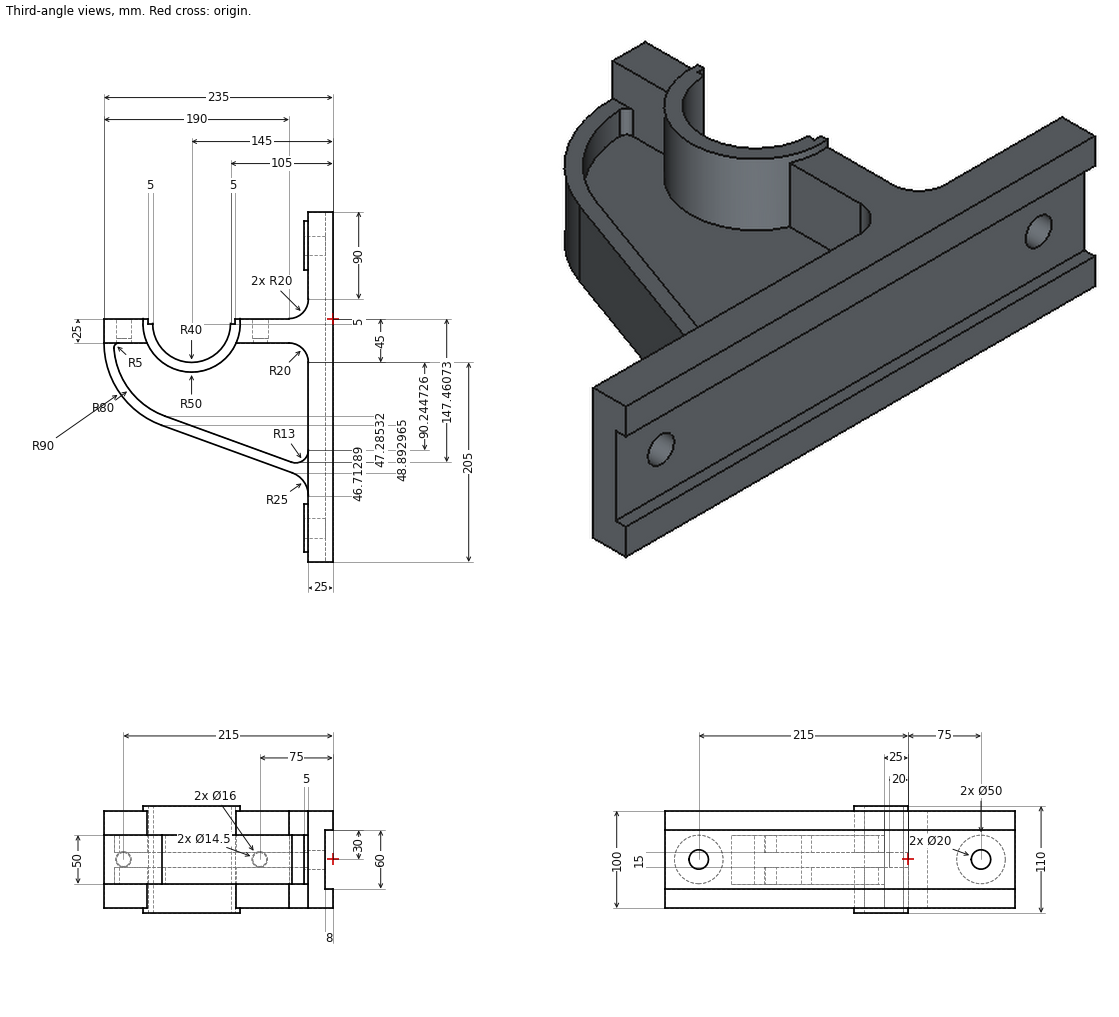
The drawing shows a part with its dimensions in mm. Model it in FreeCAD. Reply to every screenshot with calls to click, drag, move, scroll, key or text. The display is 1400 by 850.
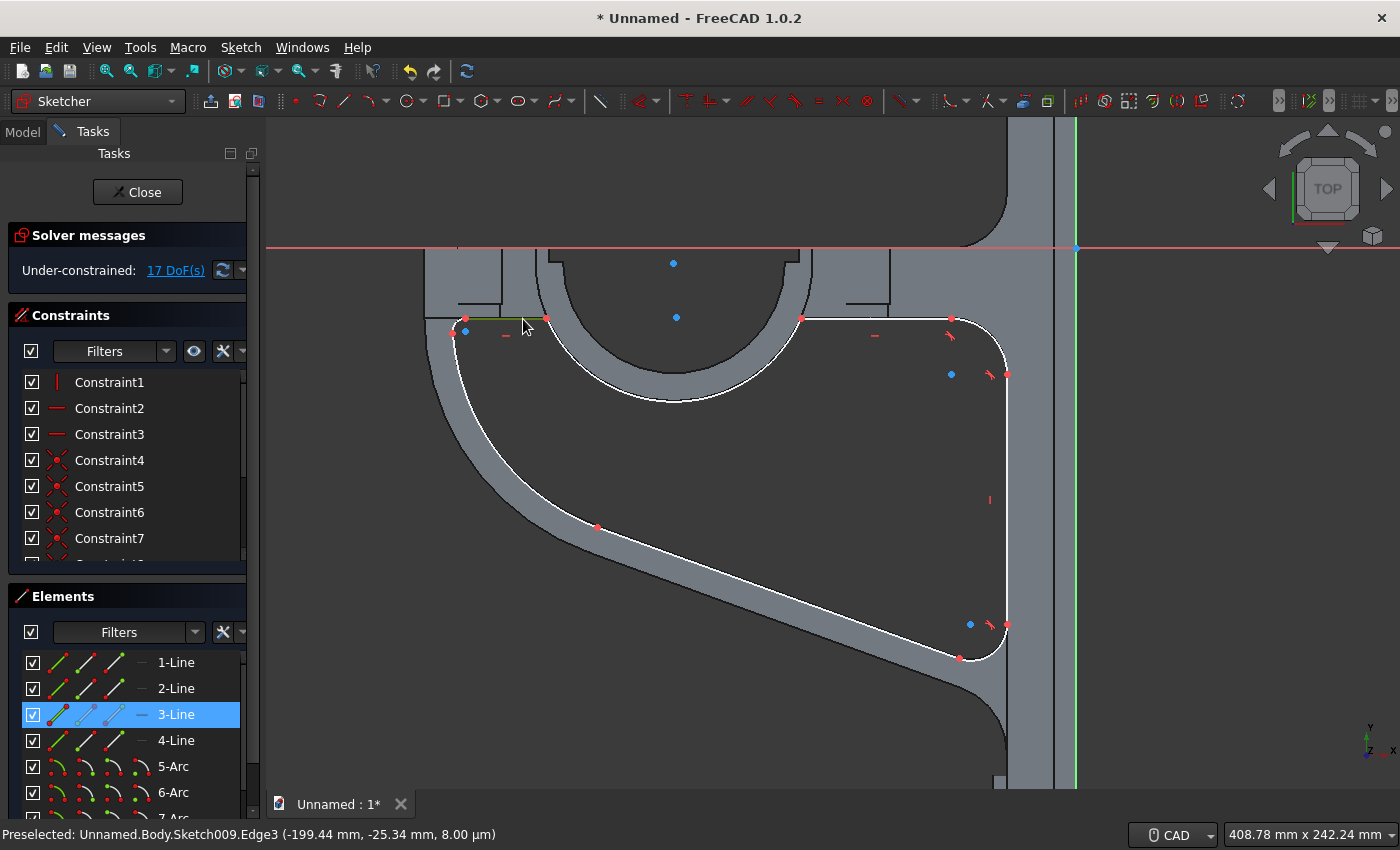
scroll(456, 323, up, 2)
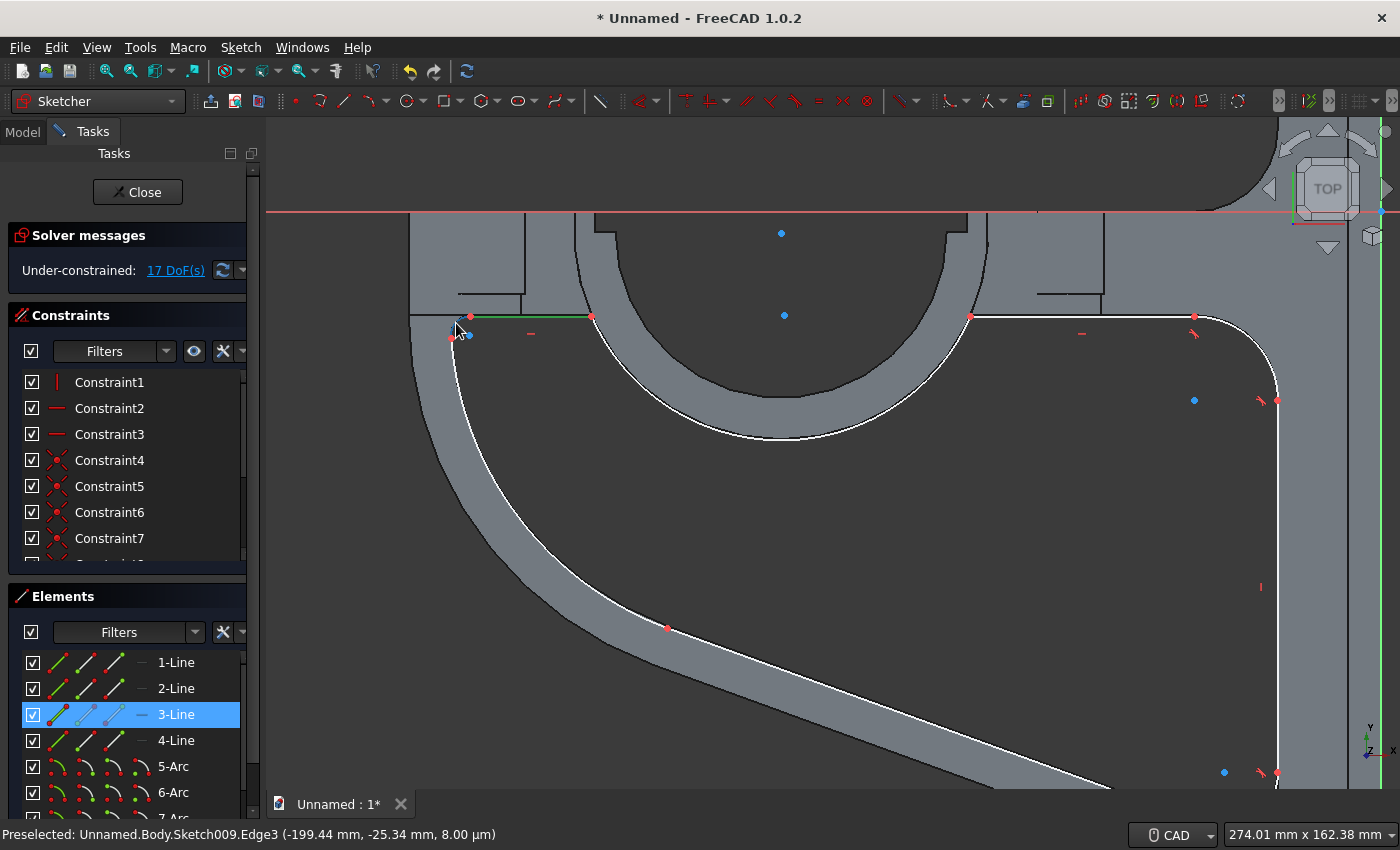
click(456, 323)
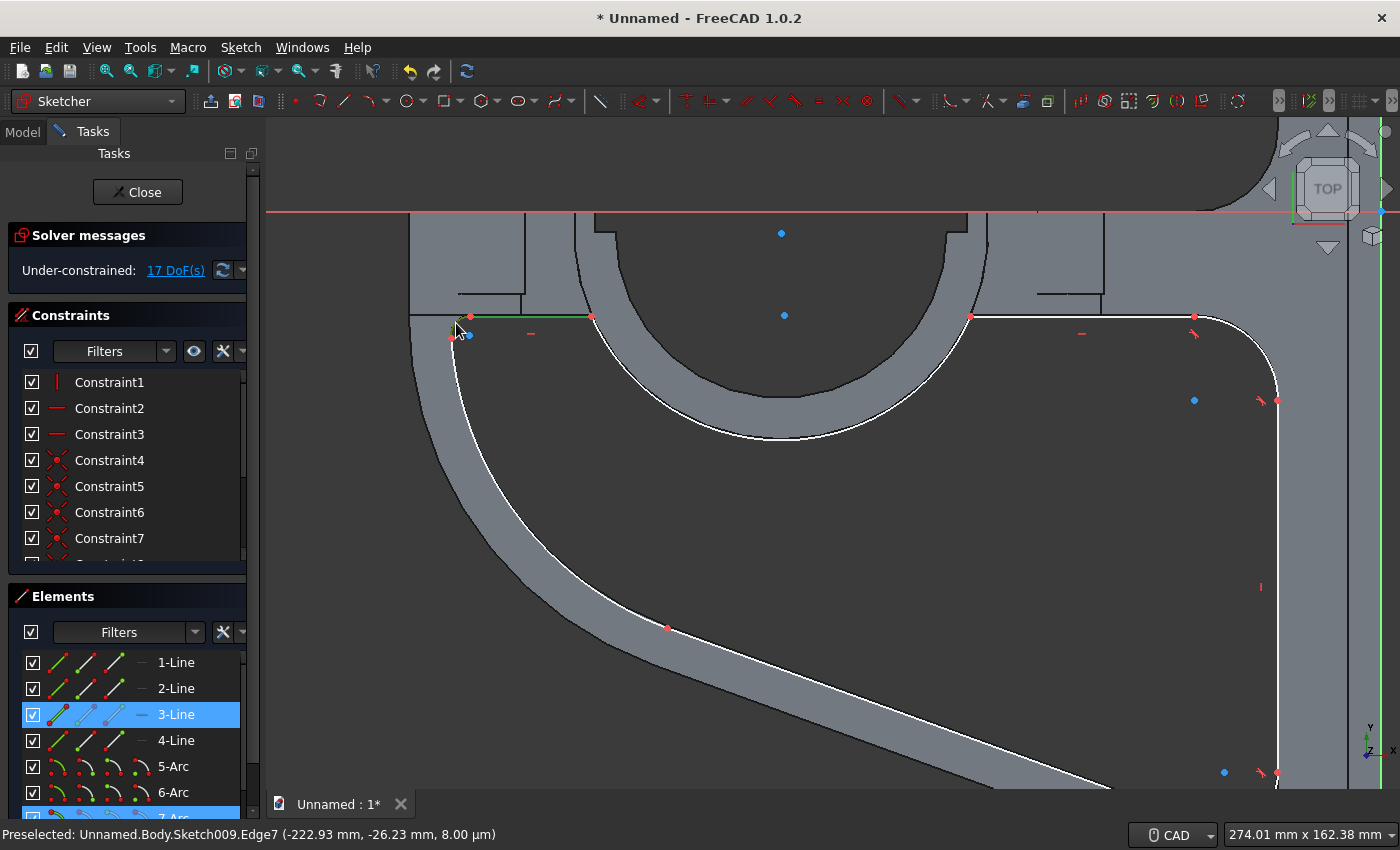
click(796, 102)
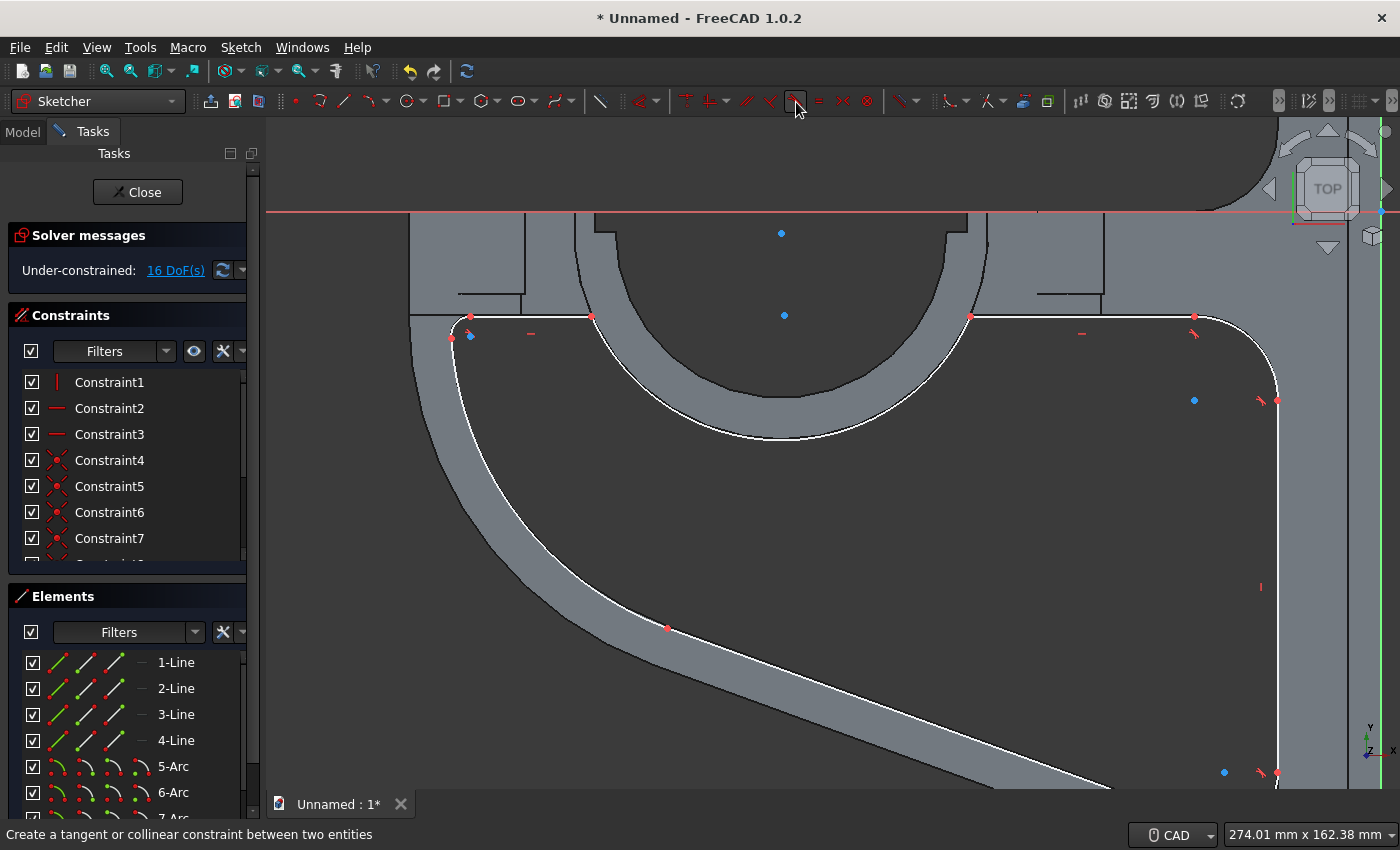
click(829, 687)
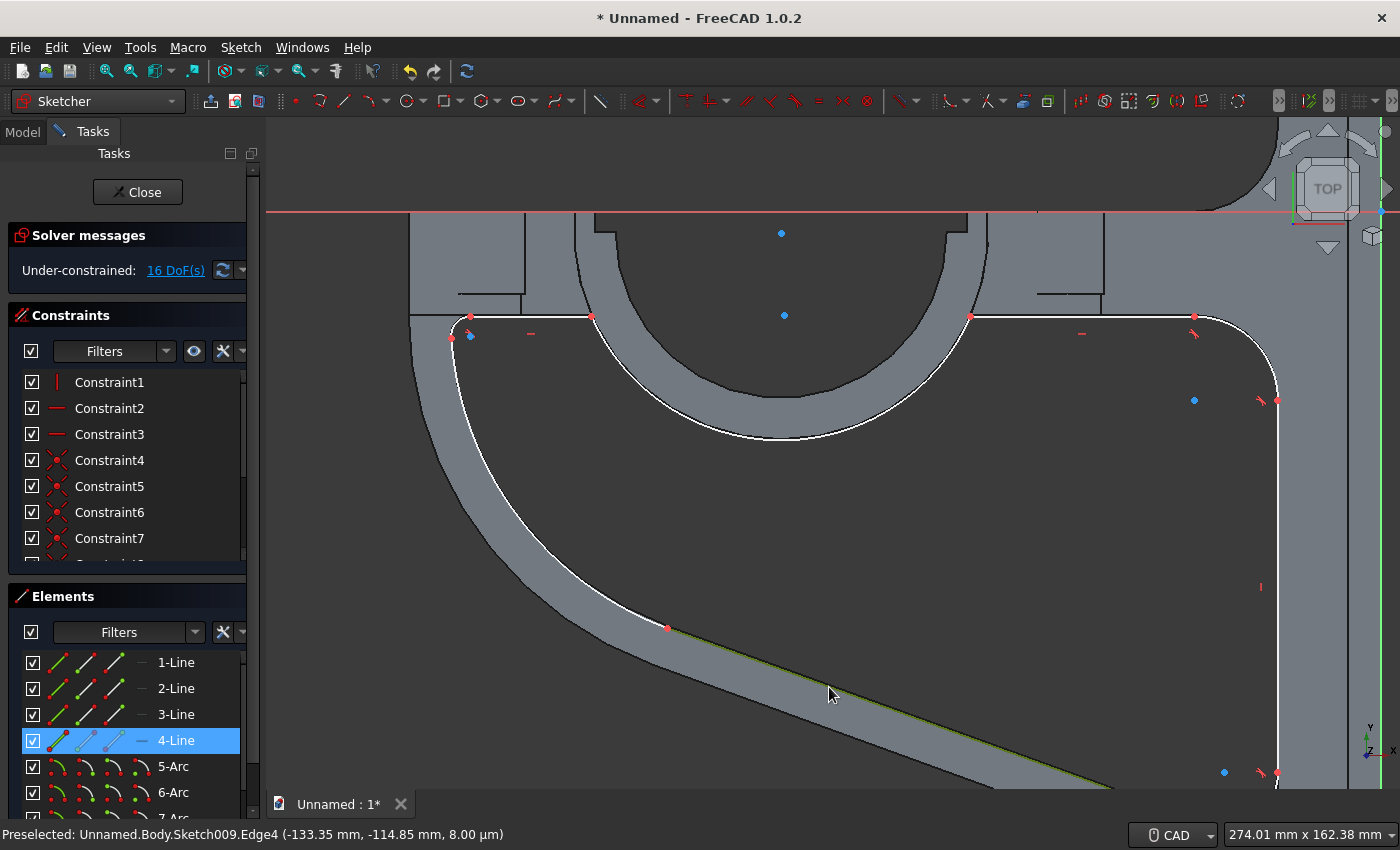
scroll(456, 323, down, 2)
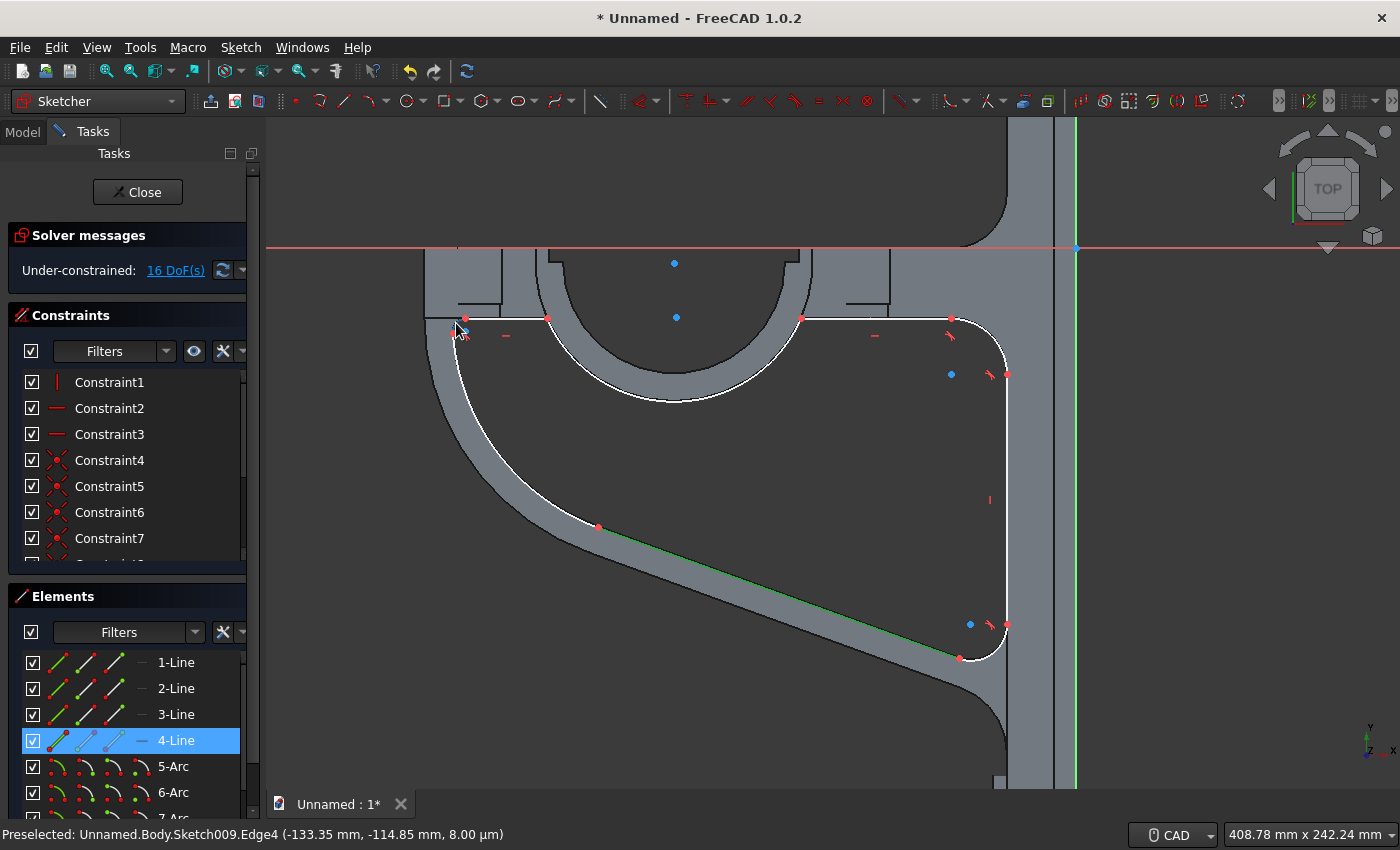
click(979, 660)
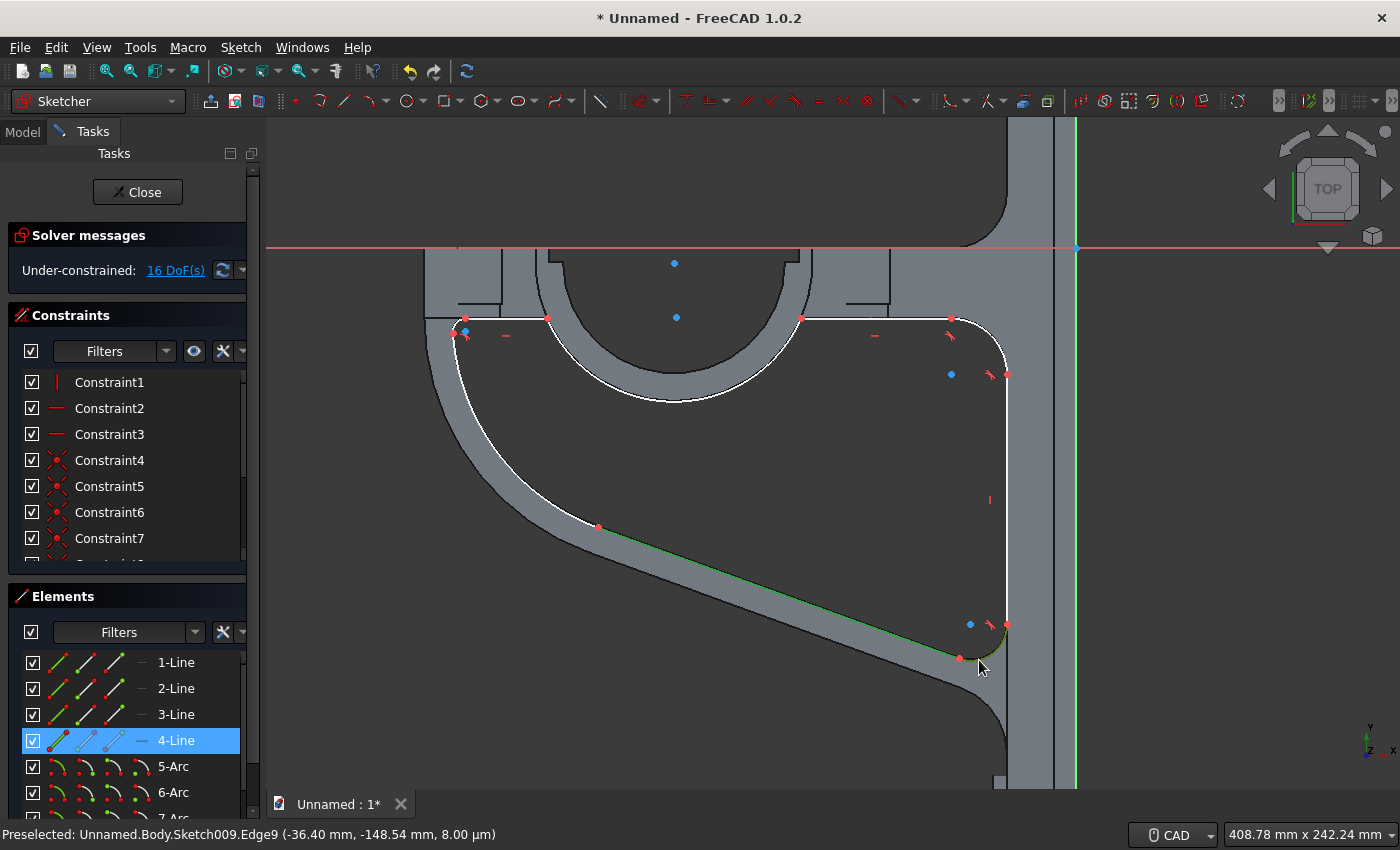
click(796, 102)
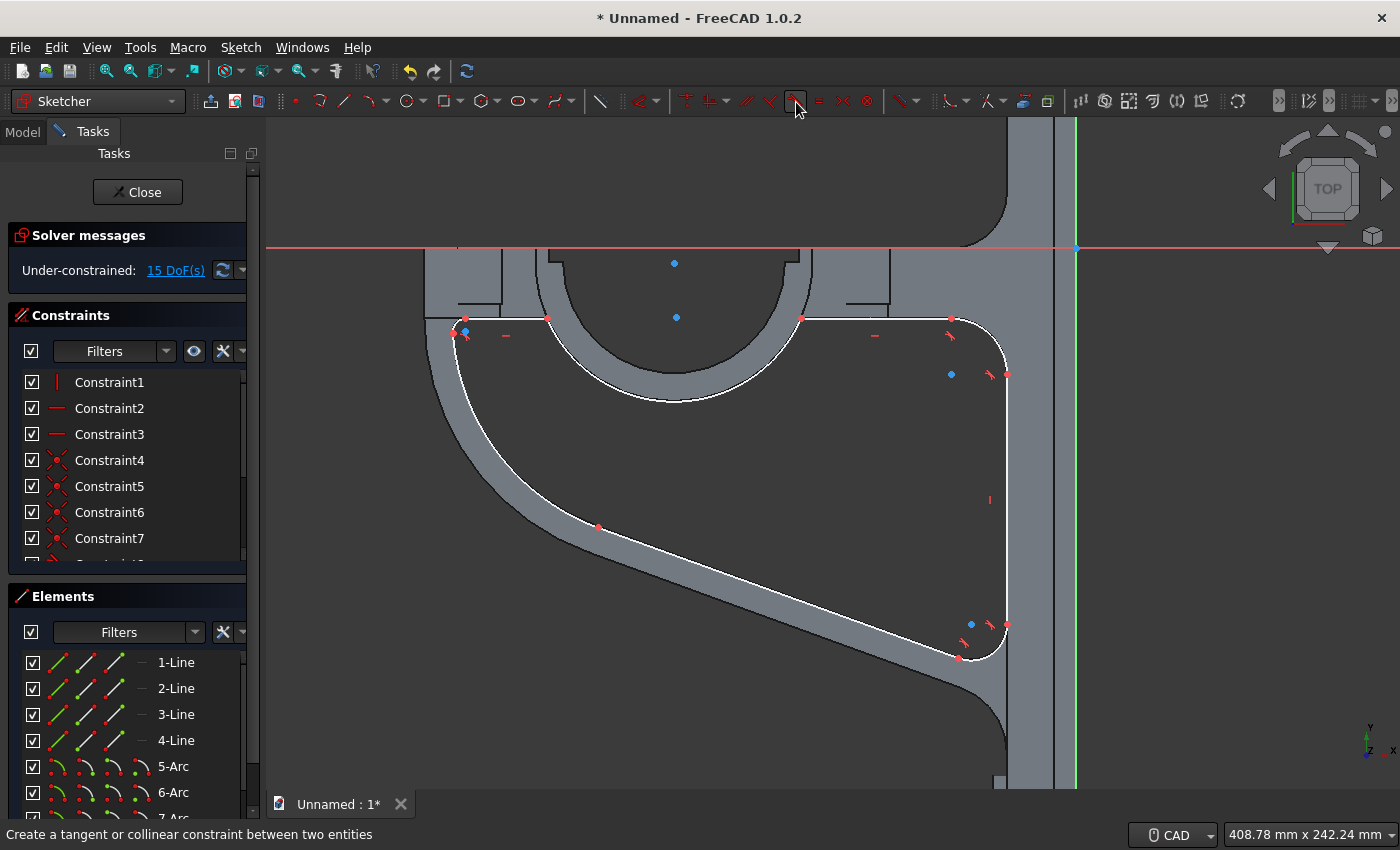
scroll(456, 323, up, 2)